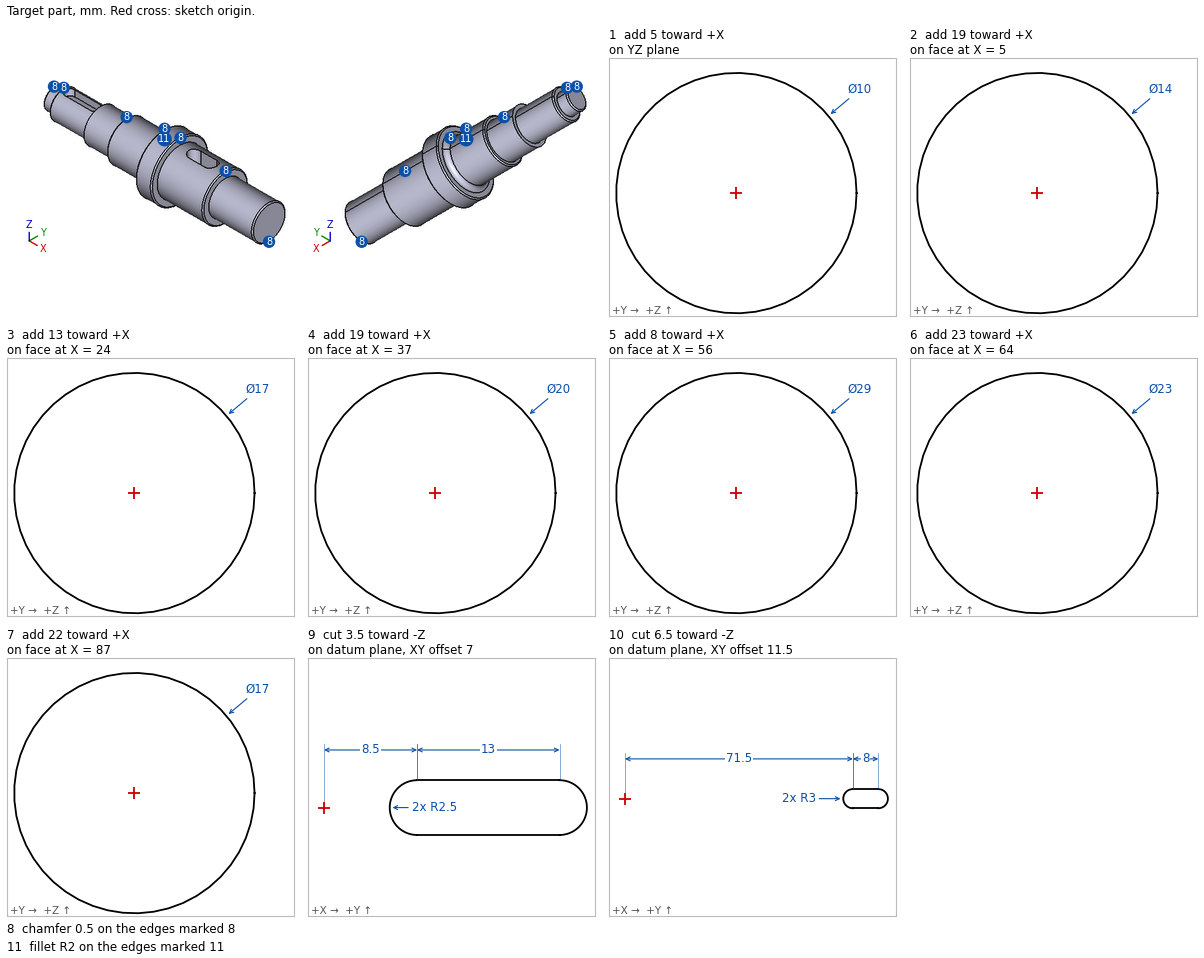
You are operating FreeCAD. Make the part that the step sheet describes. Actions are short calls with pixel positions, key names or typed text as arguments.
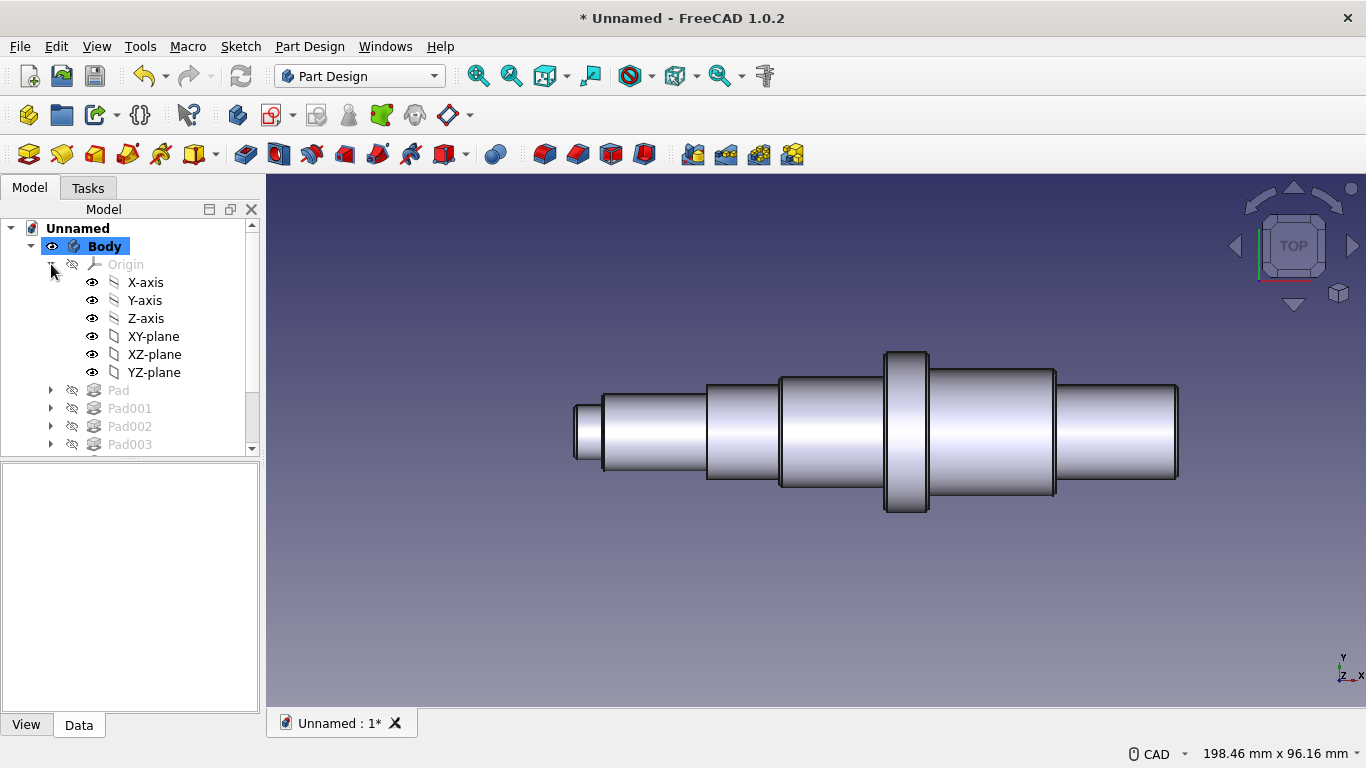
click(137, 336)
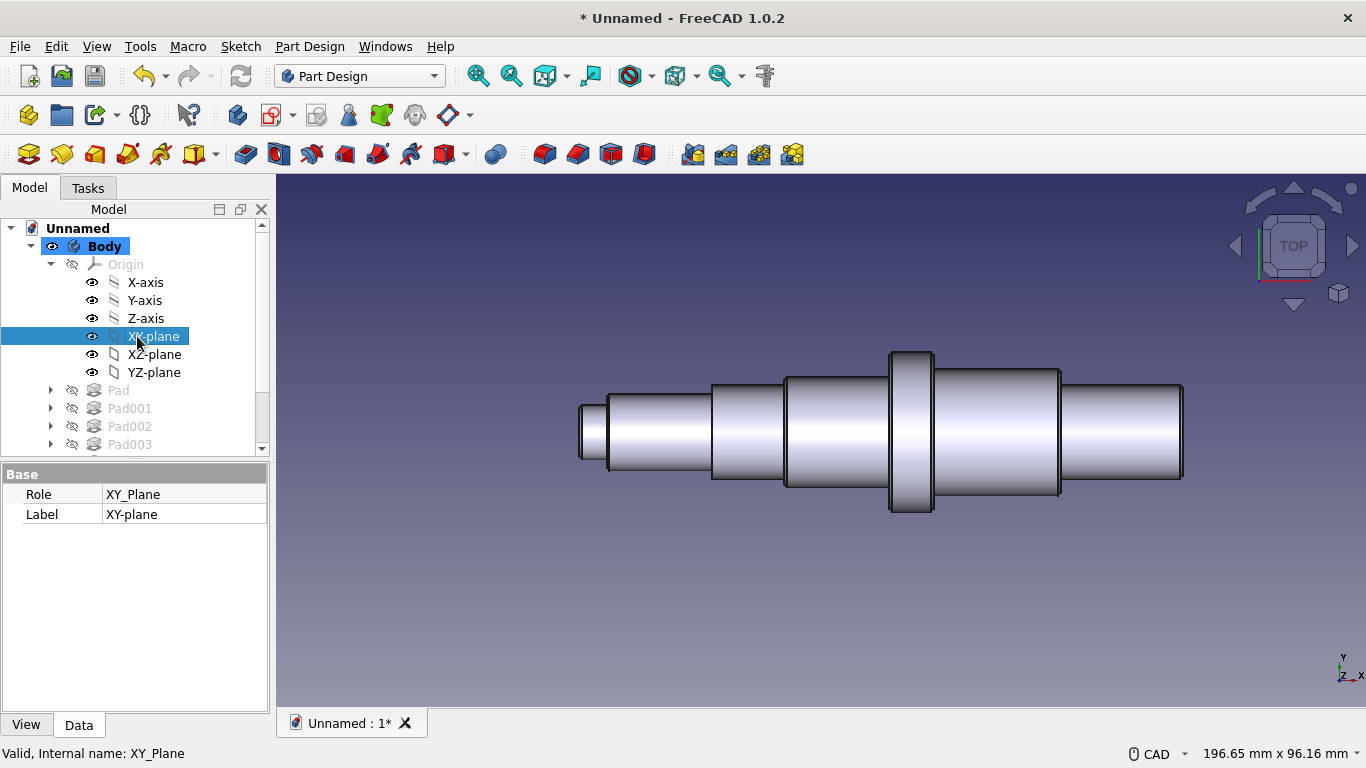
click(448, 116)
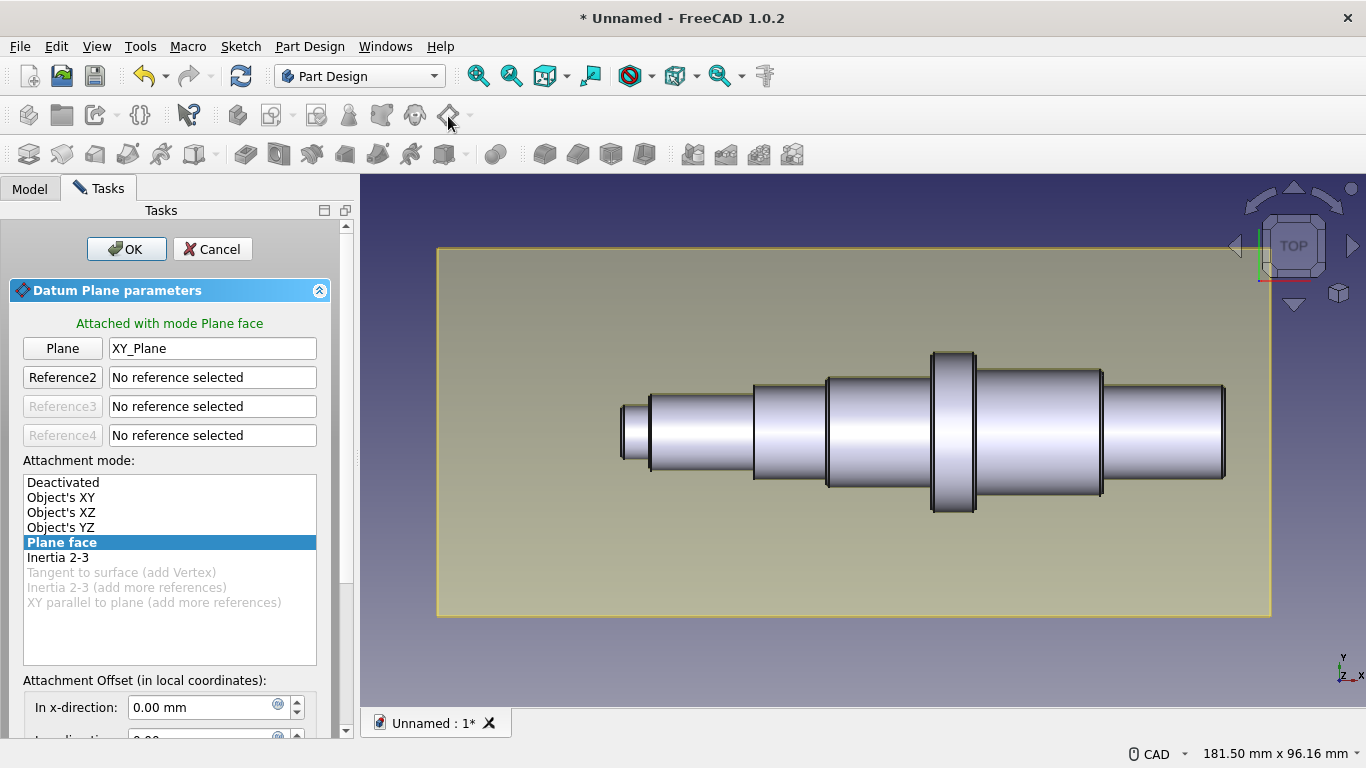
scroll(346, 479, down, 2)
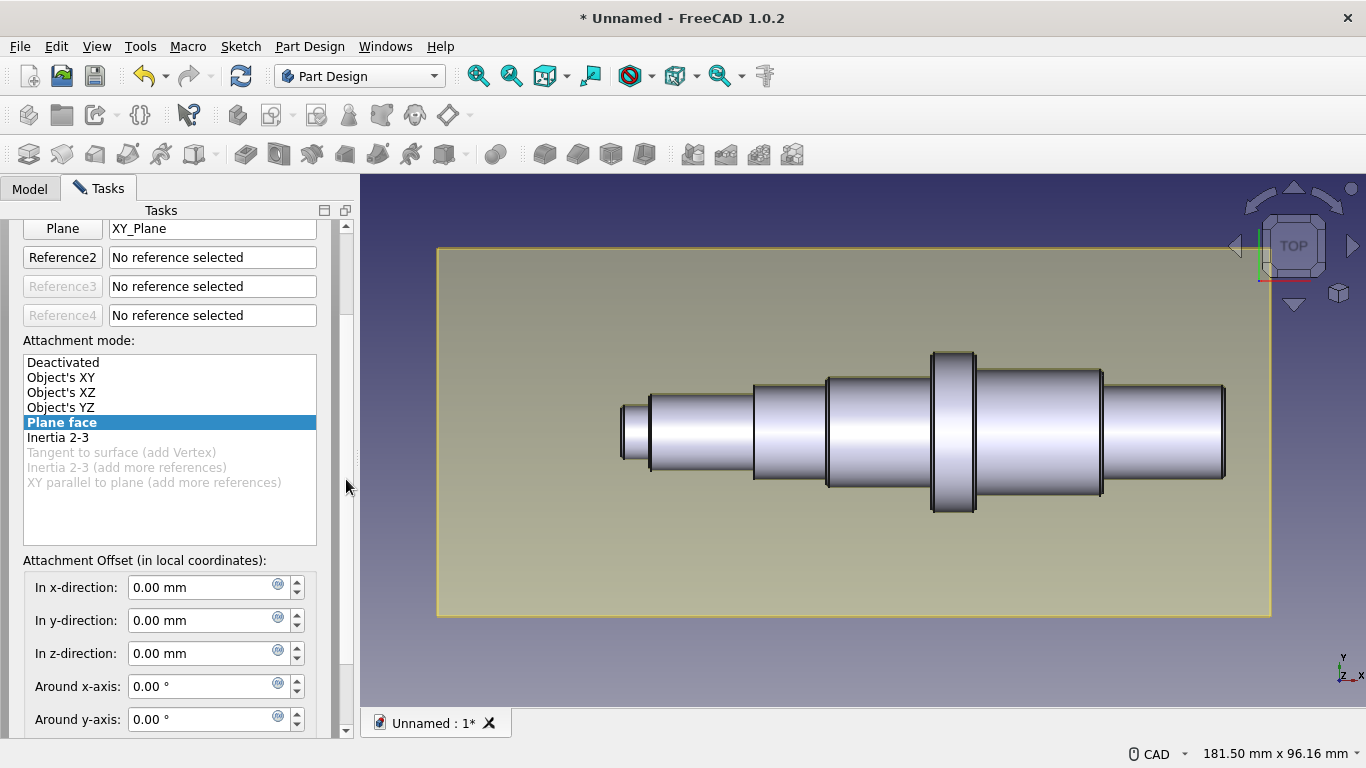
triple_click(210, 654)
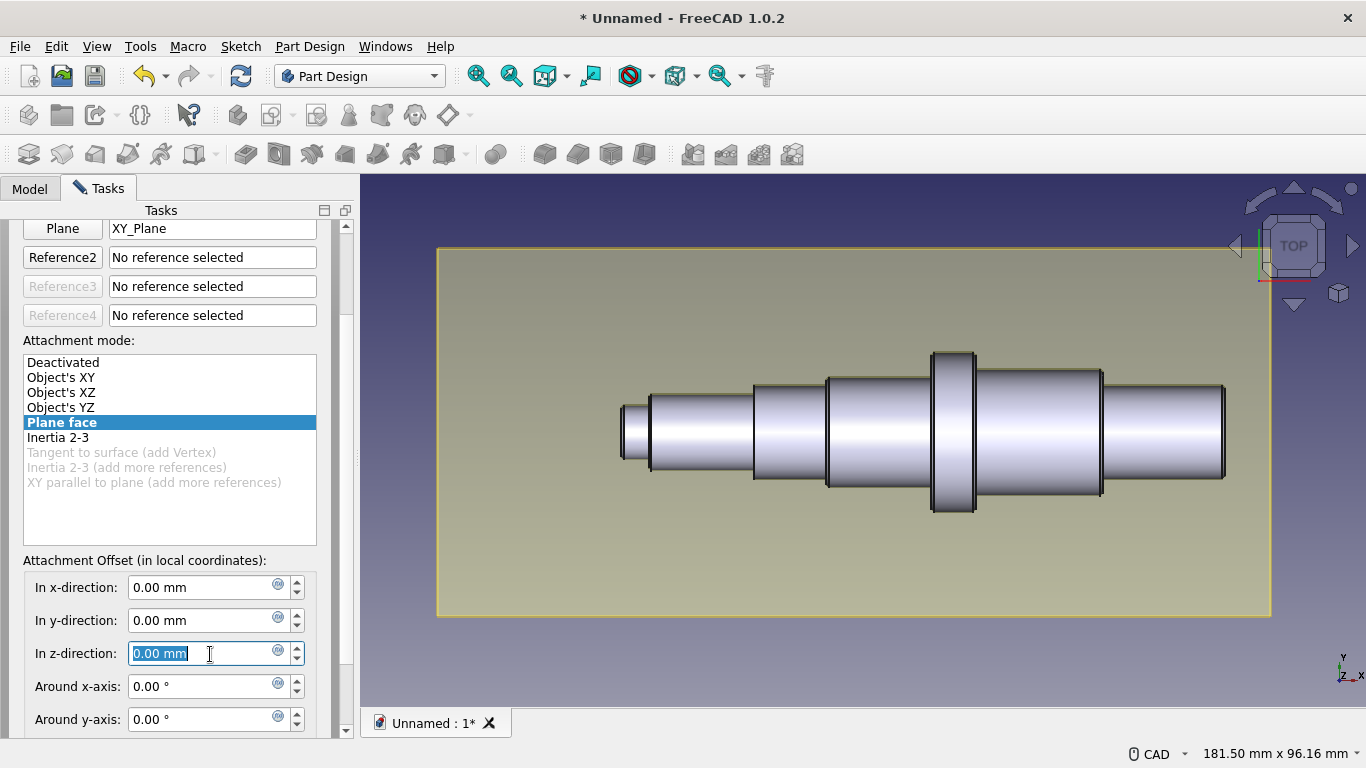
text(7)
key(Tab)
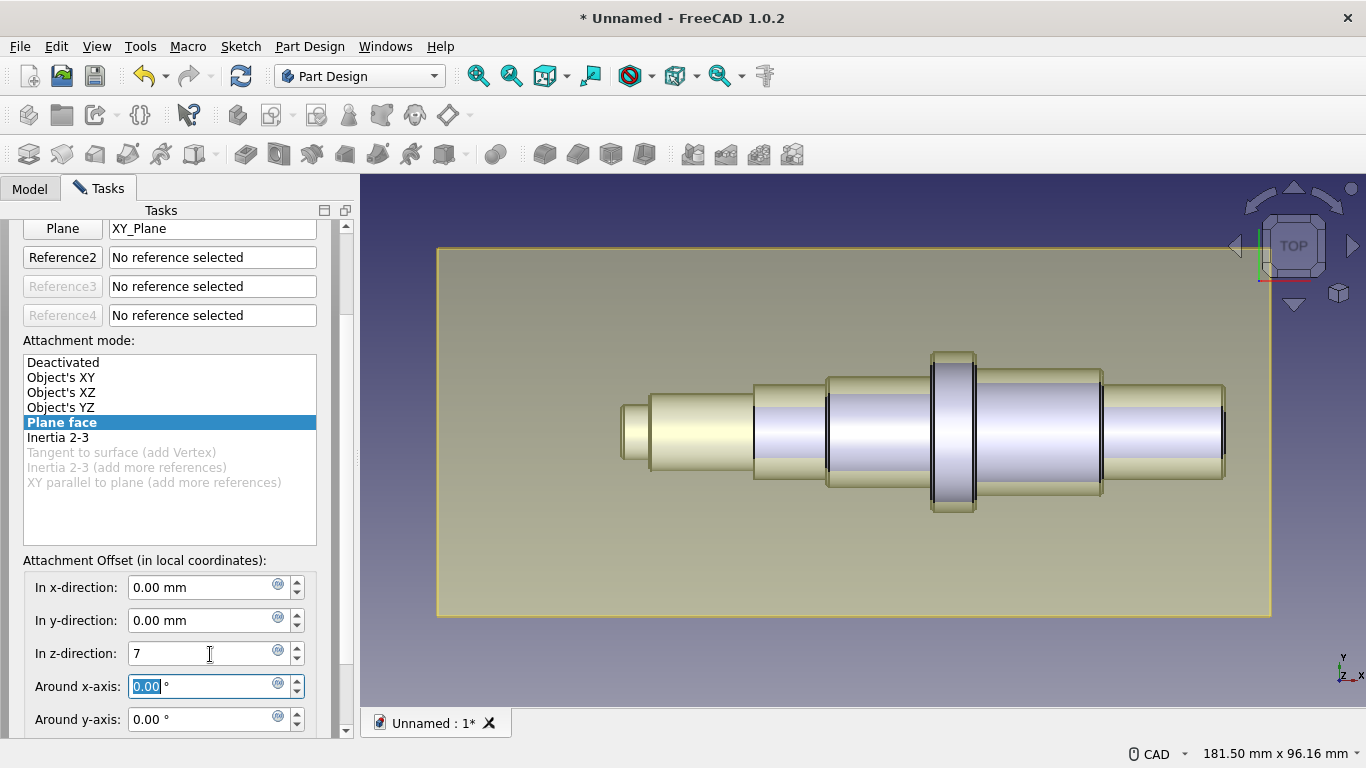
scroll(346, 479, up, 3)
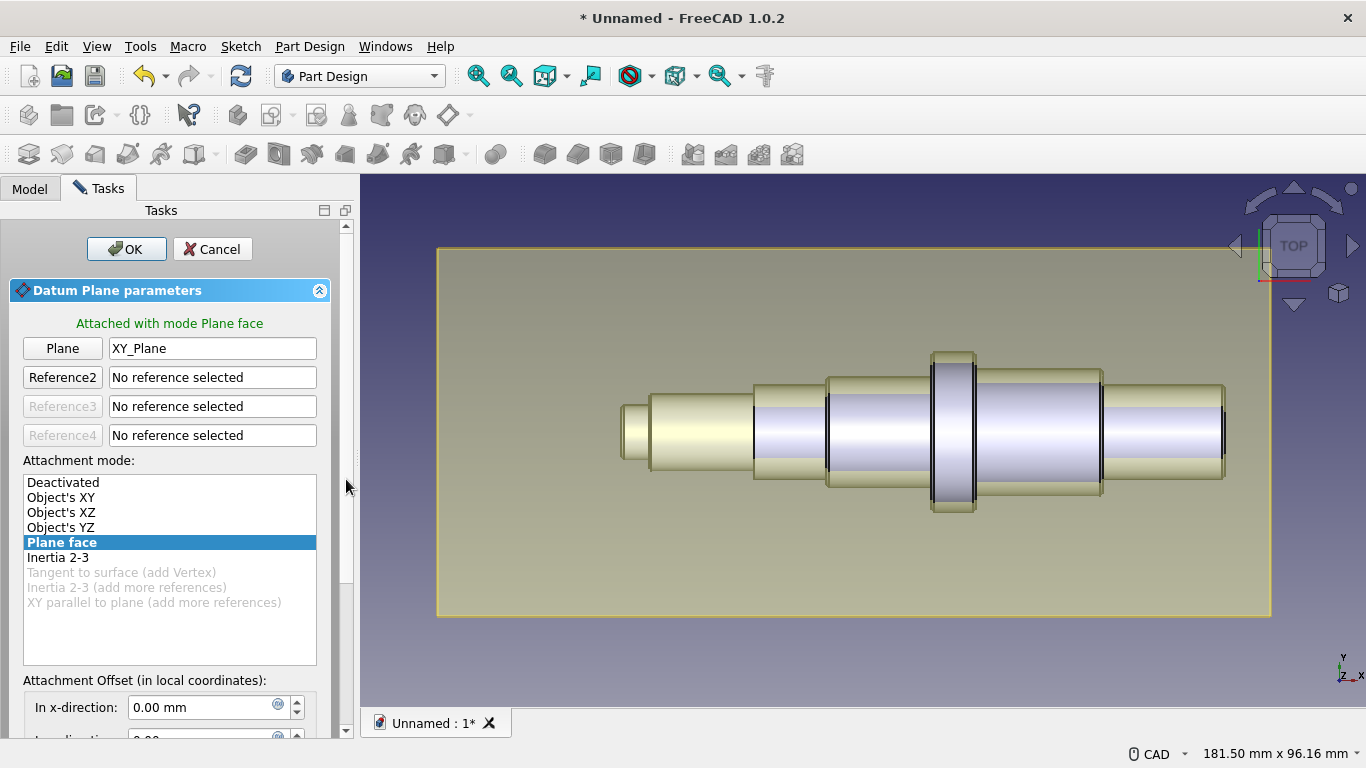
click(127, 249)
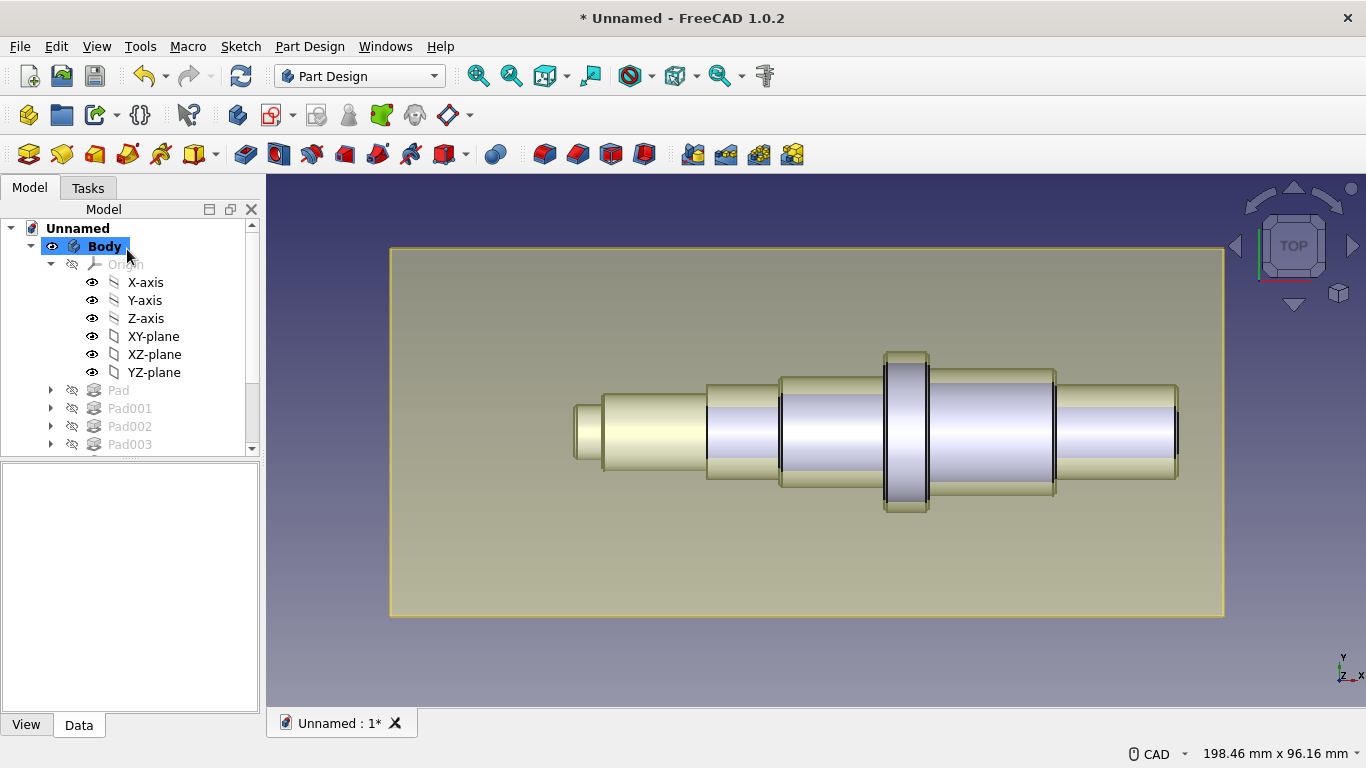
scroll(101, 332, down, 3)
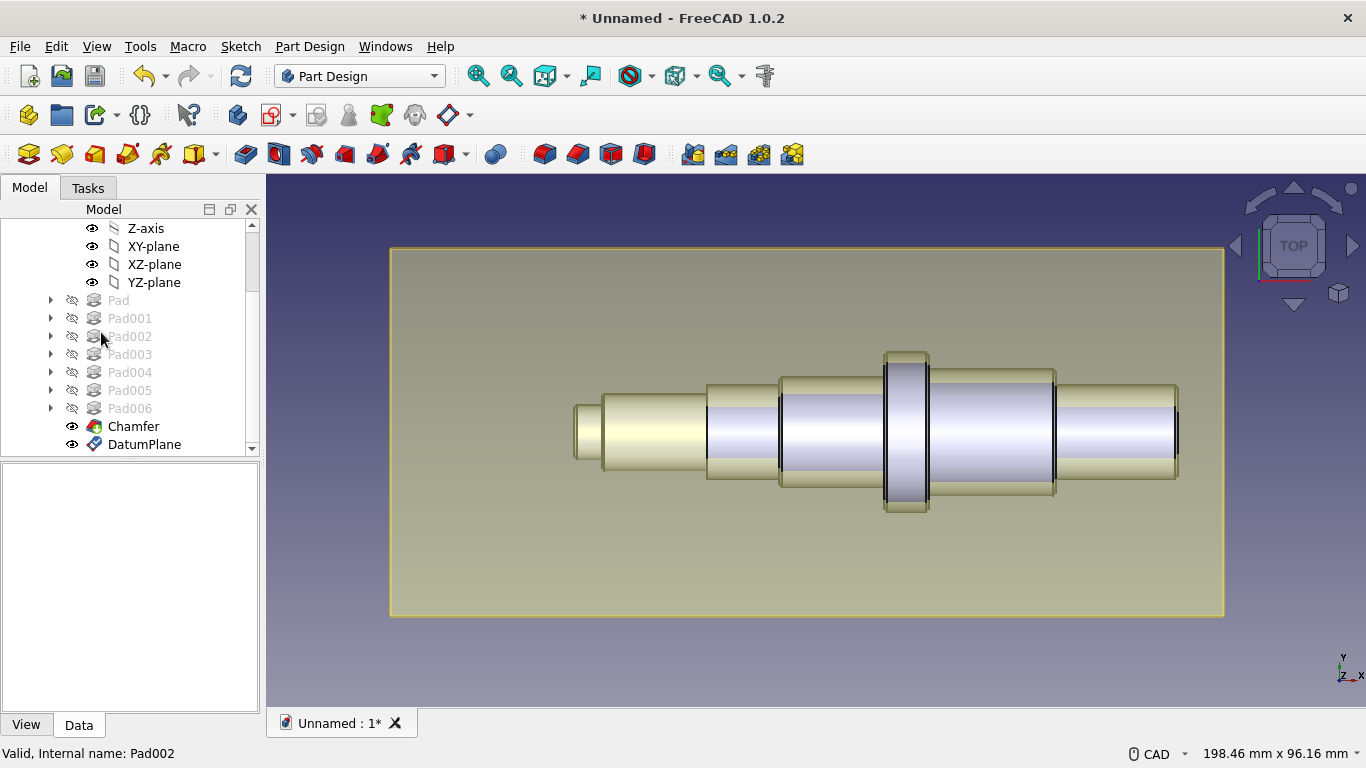
click(117, 444)